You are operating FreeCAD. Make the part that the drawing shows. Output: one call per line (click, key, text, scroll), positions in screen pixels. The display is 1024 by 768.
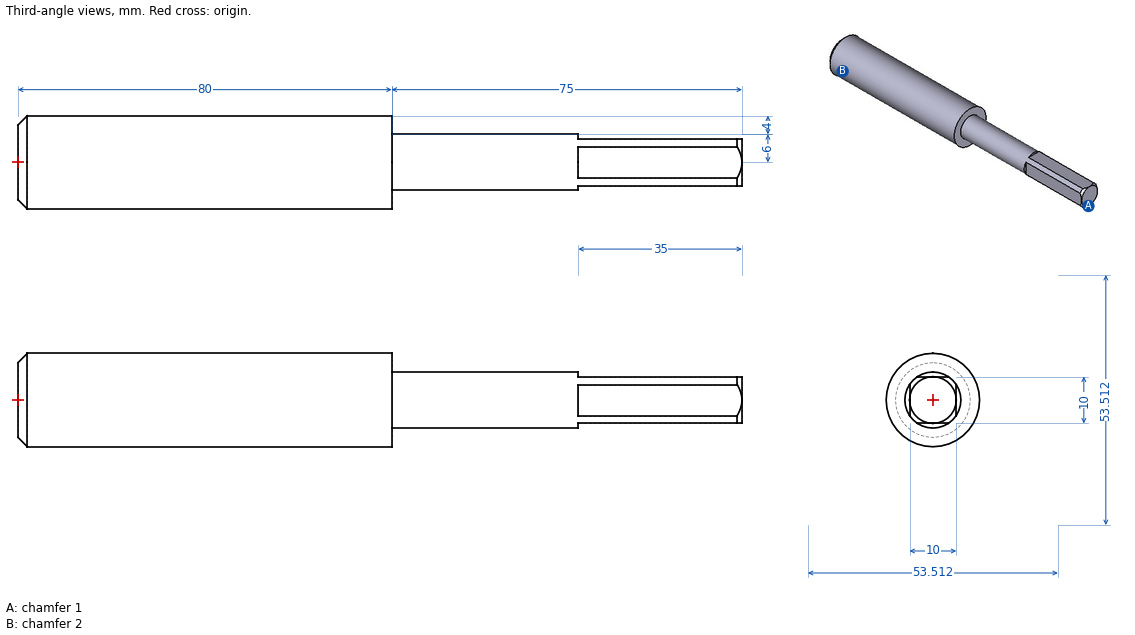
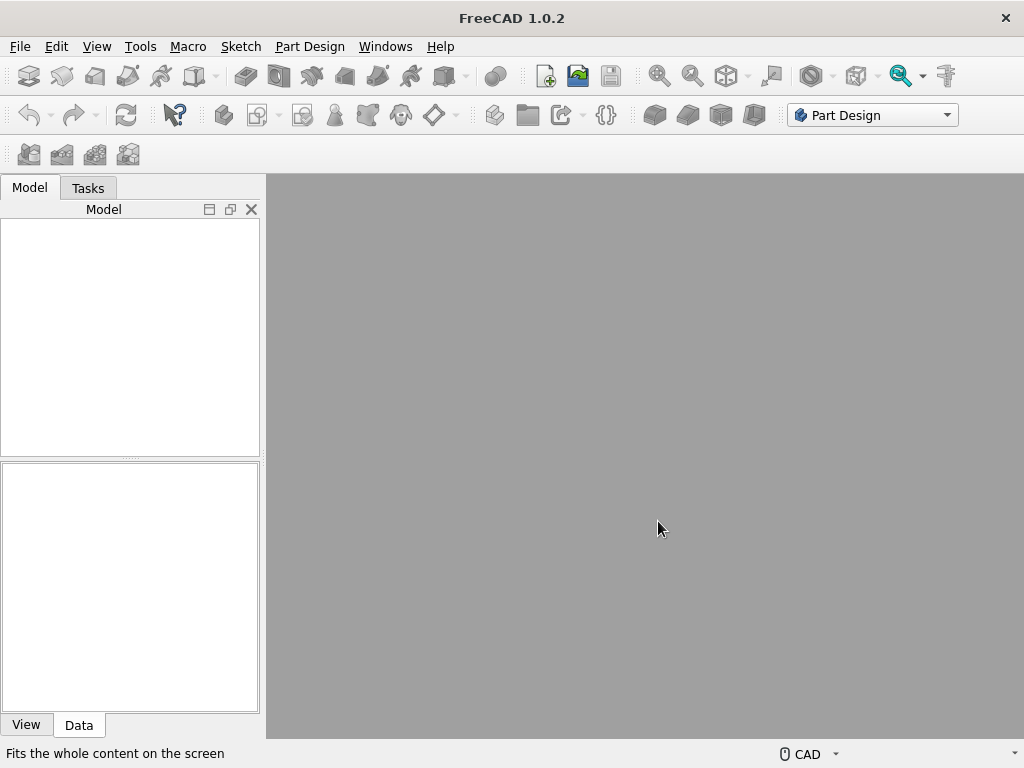
click(545, 76)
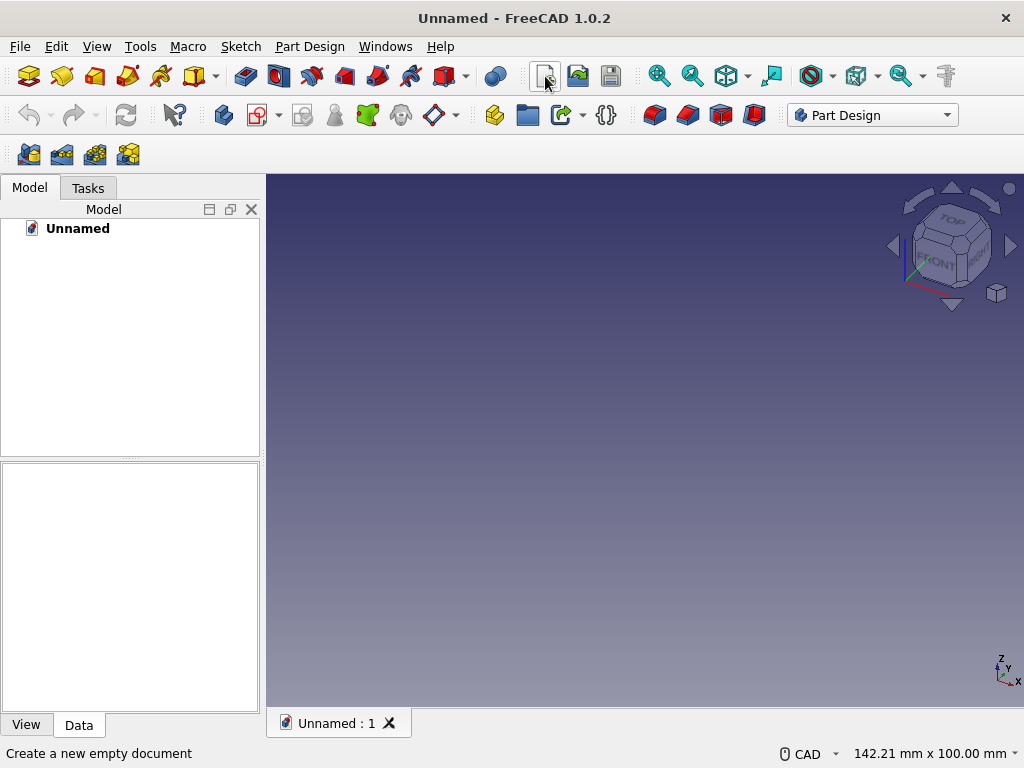
click(256, 116)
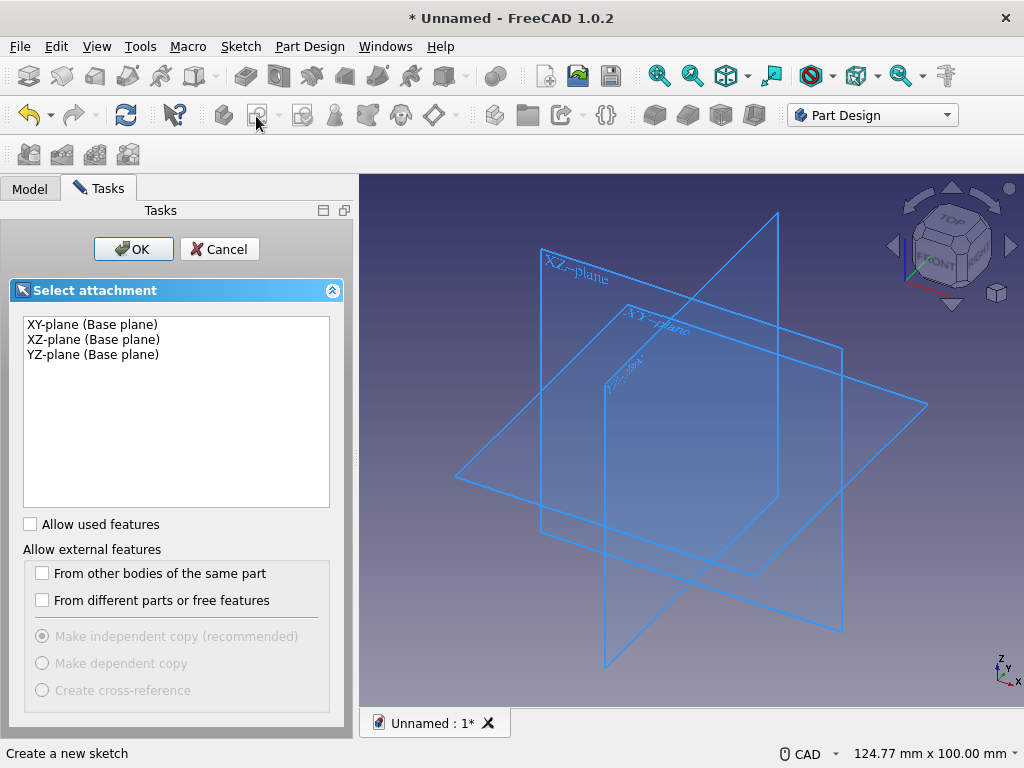
click(84, 324)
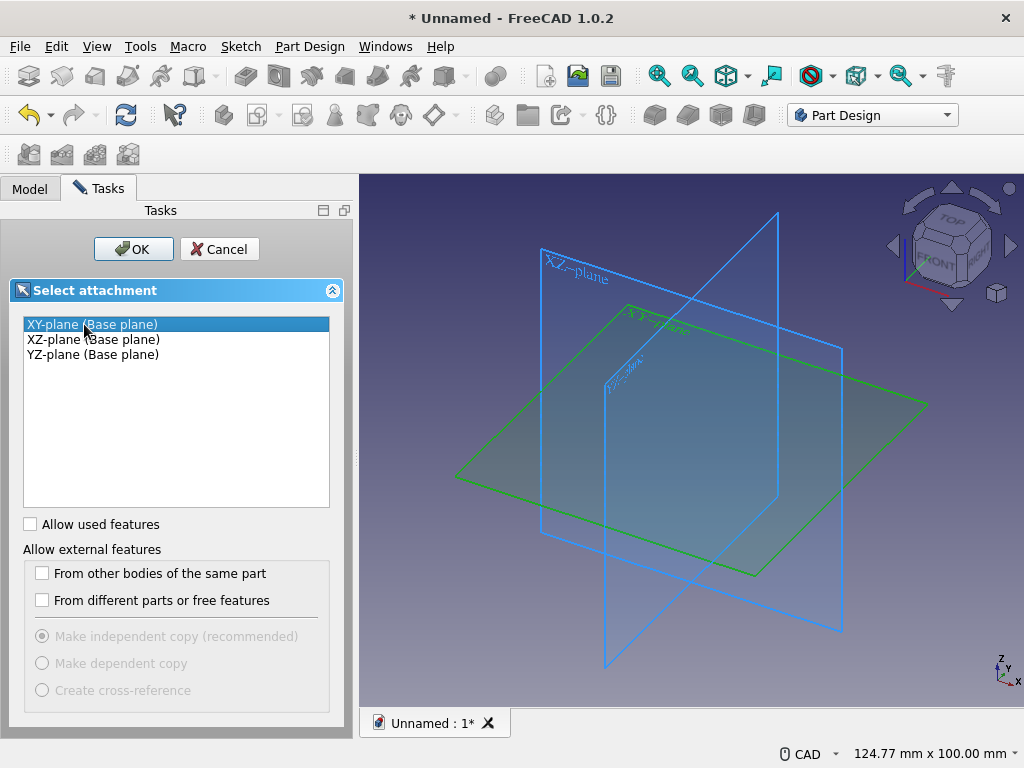
click(134, 249)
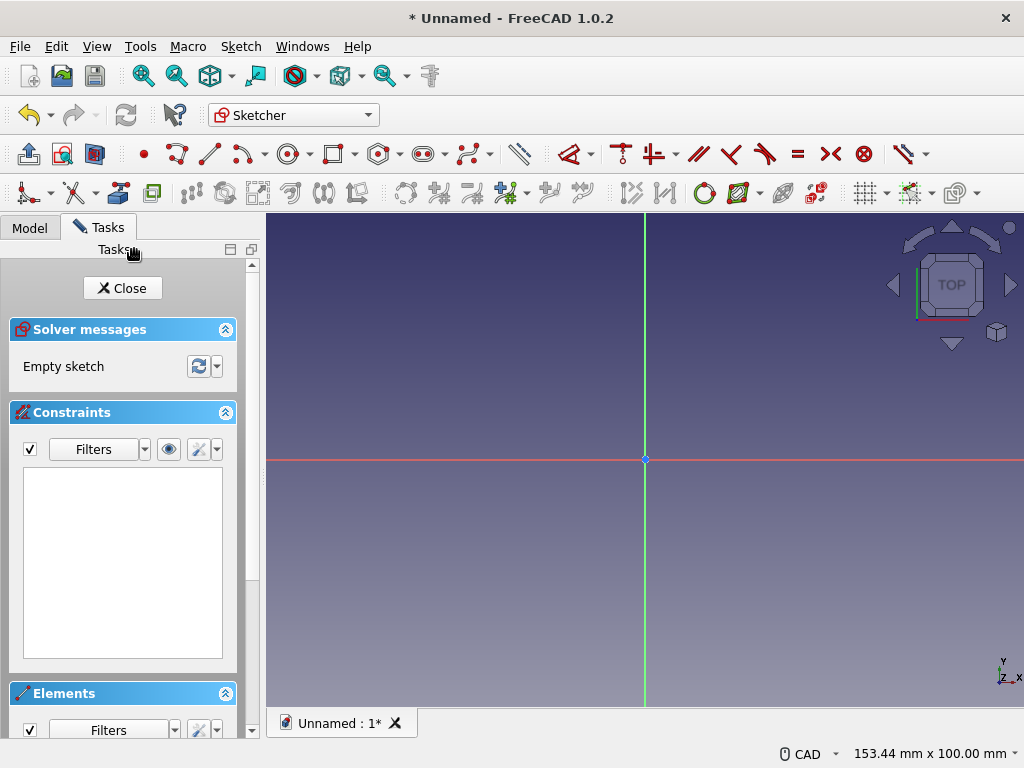
scroll(294, 480, down, 4)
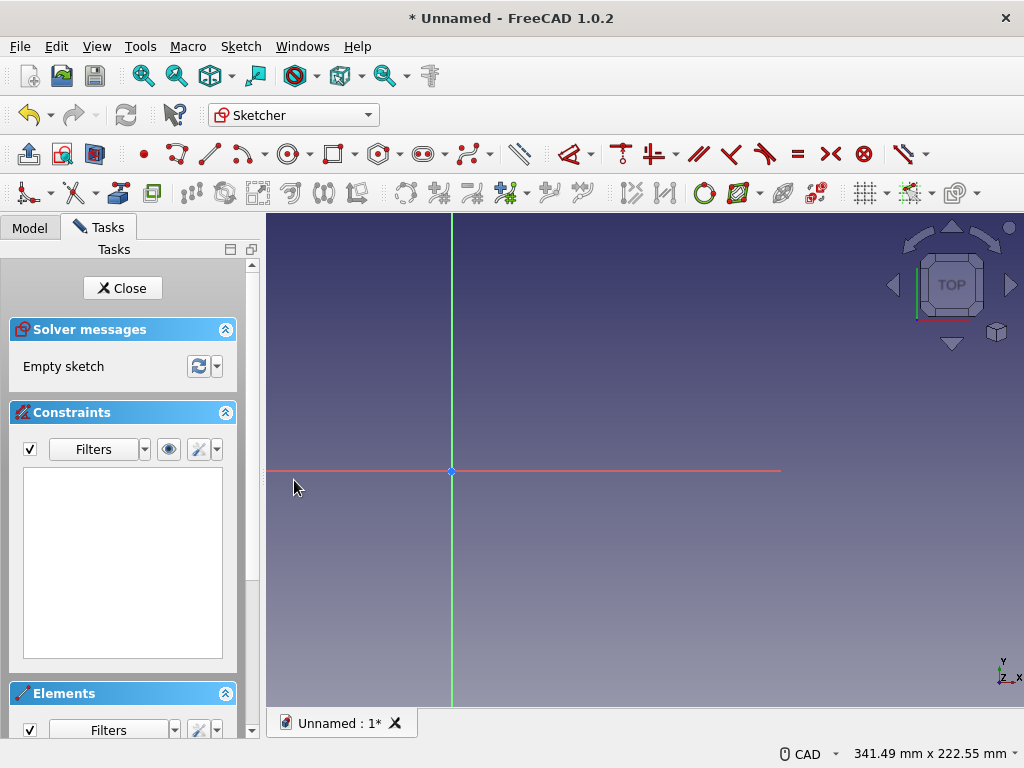
click(177, 154)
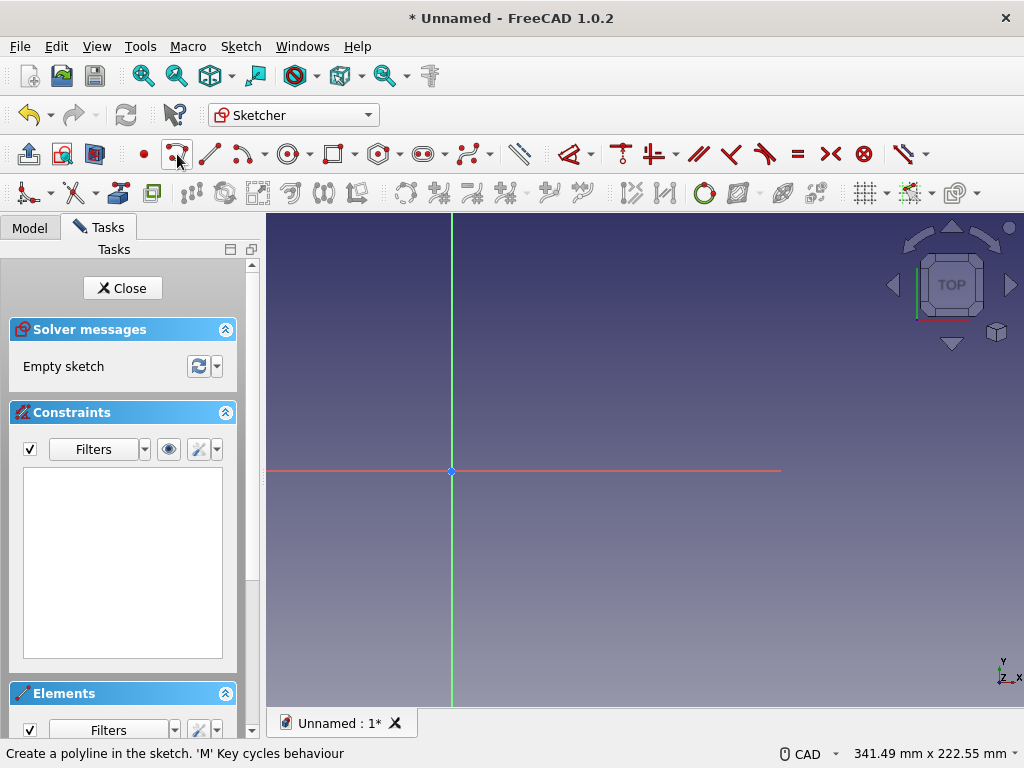
click(452, 471)
click(796, 462)
click(796, 458)
click(629, 458)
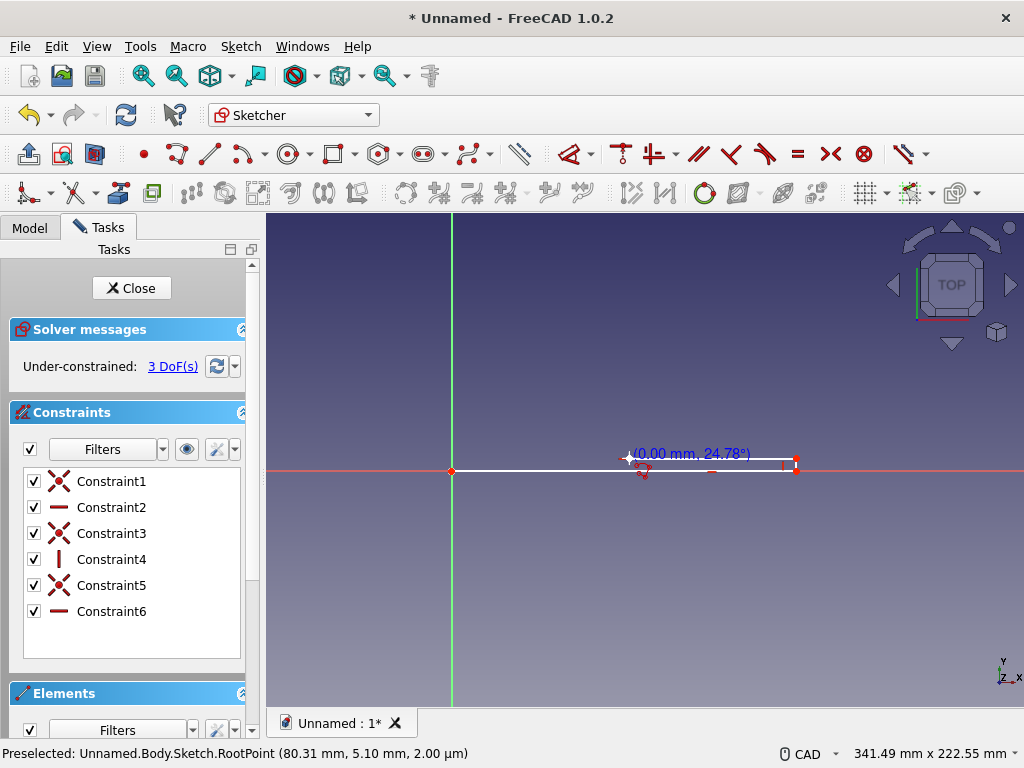
scroll(629, 449, up, 3)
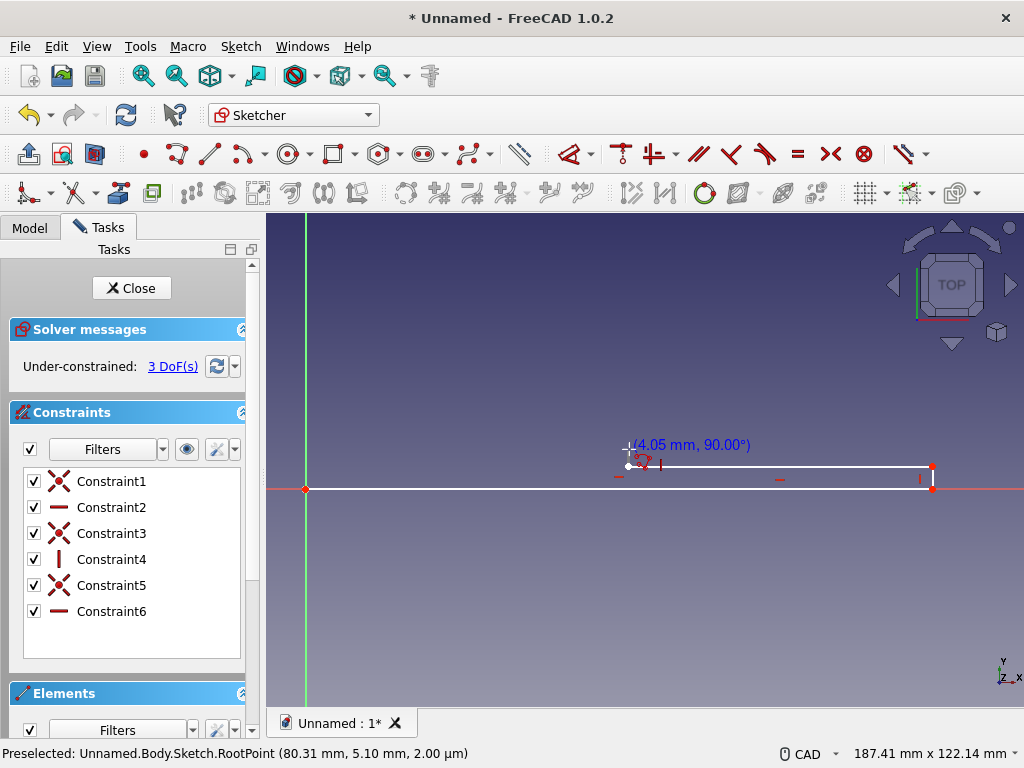
click(629, 449)
click(315, 449)
click(306, 489)
key(Escape)
key(Escape)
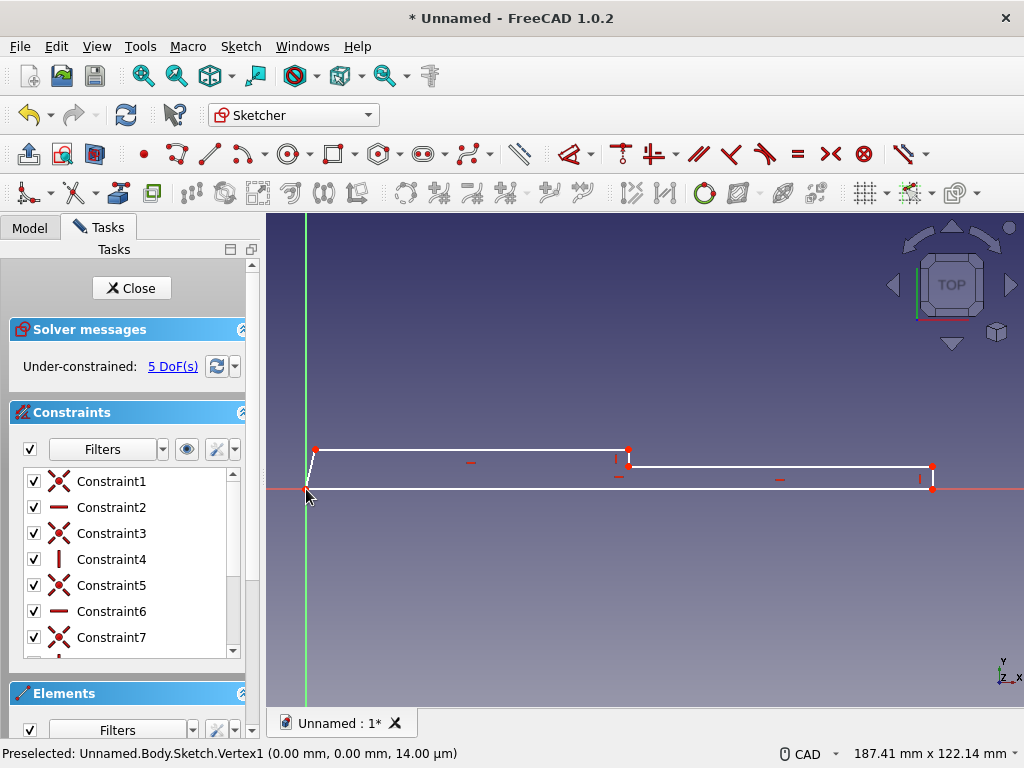
click(308, 477)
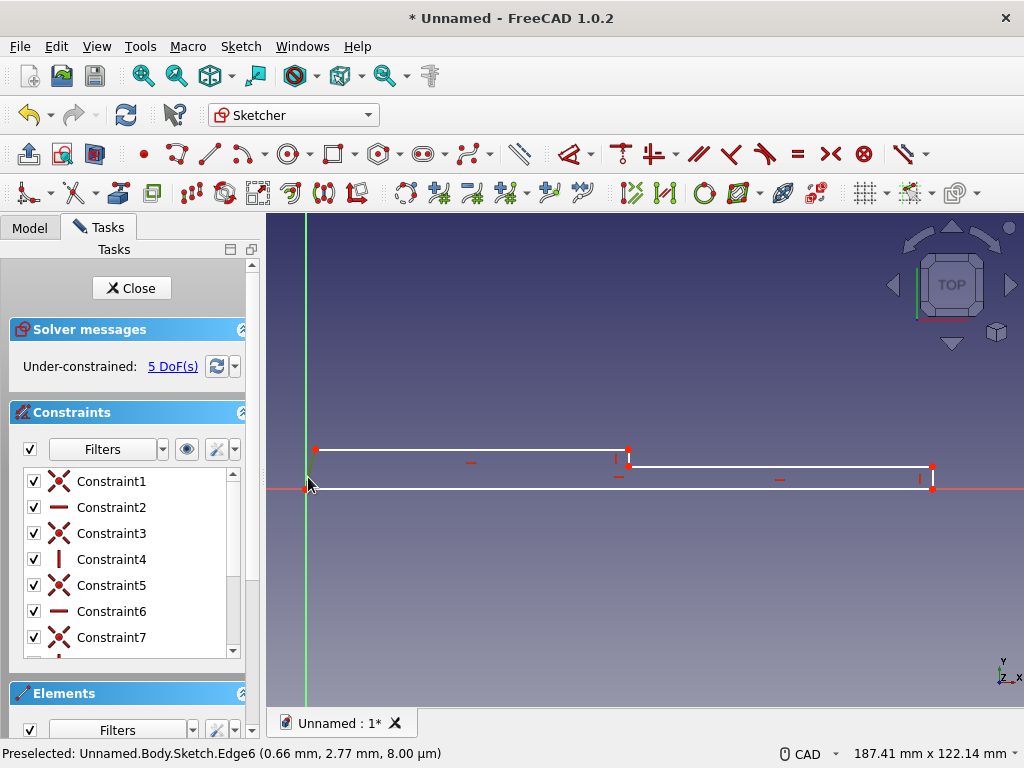
click(676, 154)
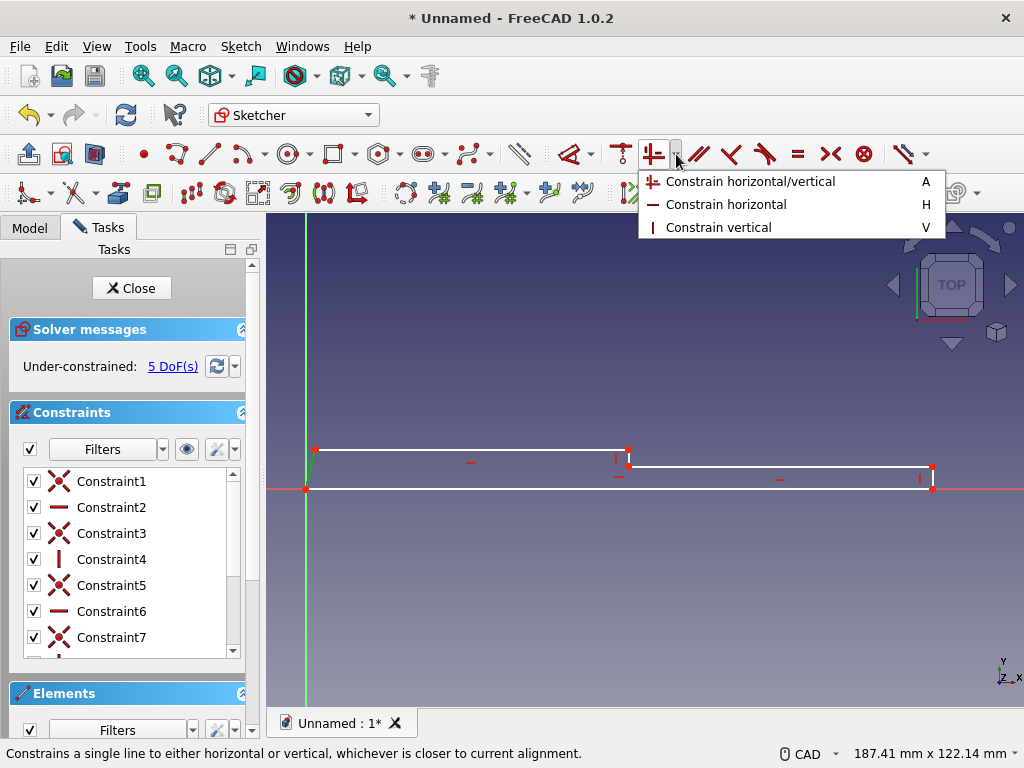
click(792, 228)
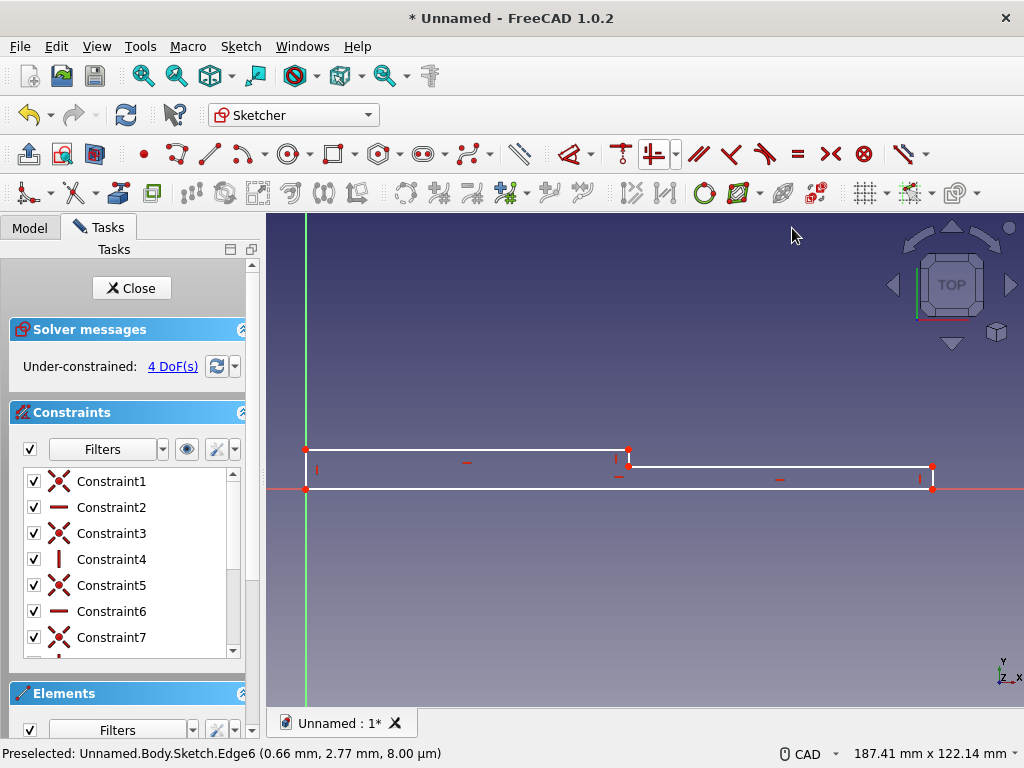
click(568, 154)